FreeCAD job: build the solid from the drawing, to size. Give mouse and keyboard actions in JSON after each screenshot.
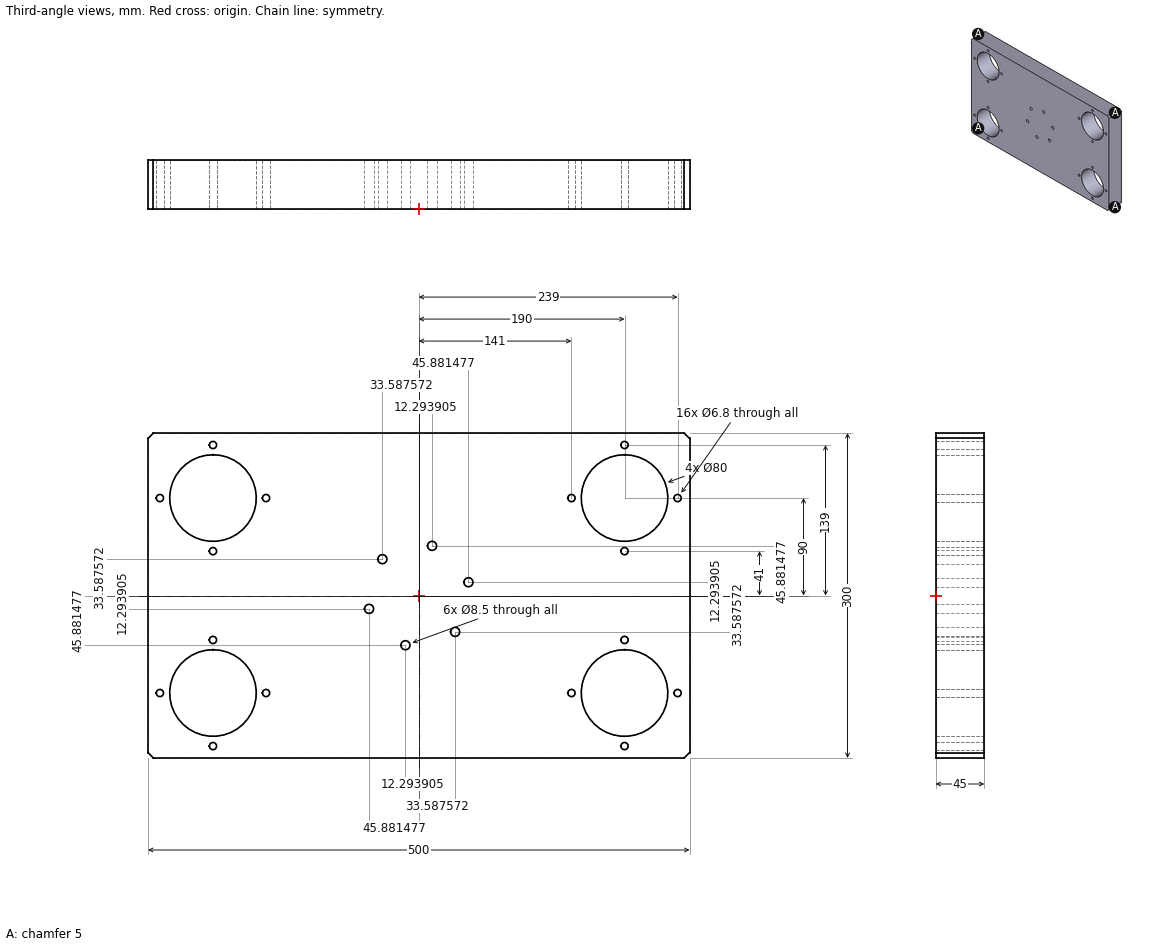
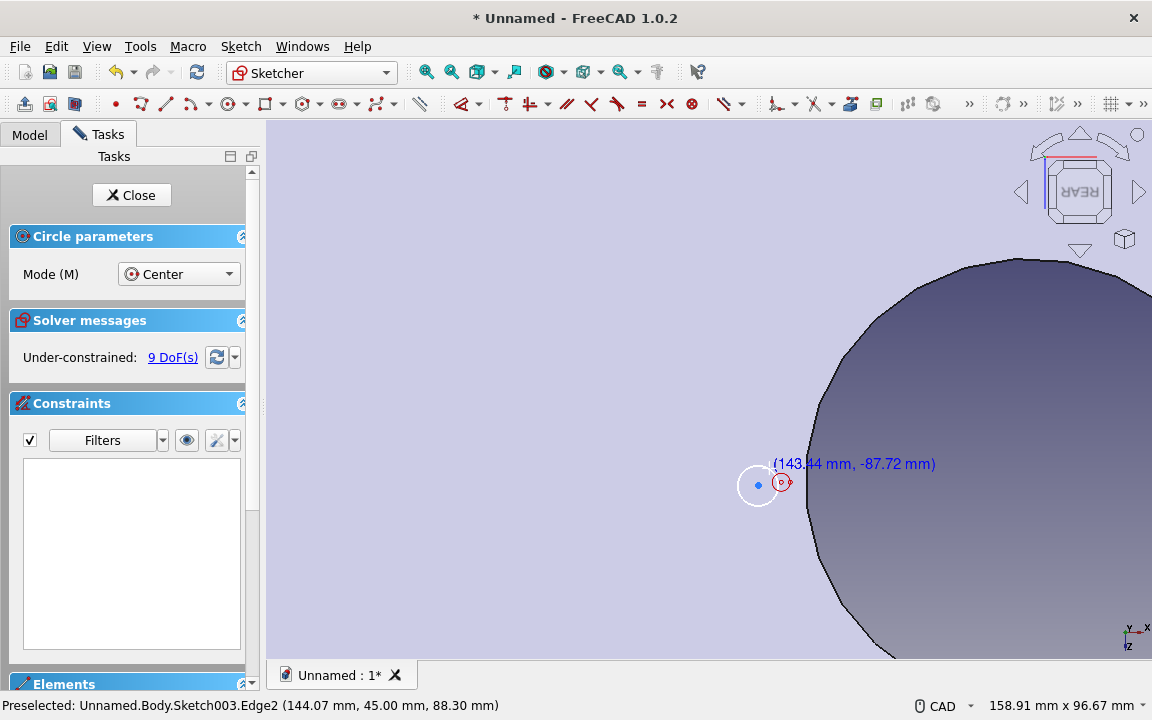
{"action": "scroll", "coordinate": [773, 471], "scroll_direction": "down", "scroll_amount": 9}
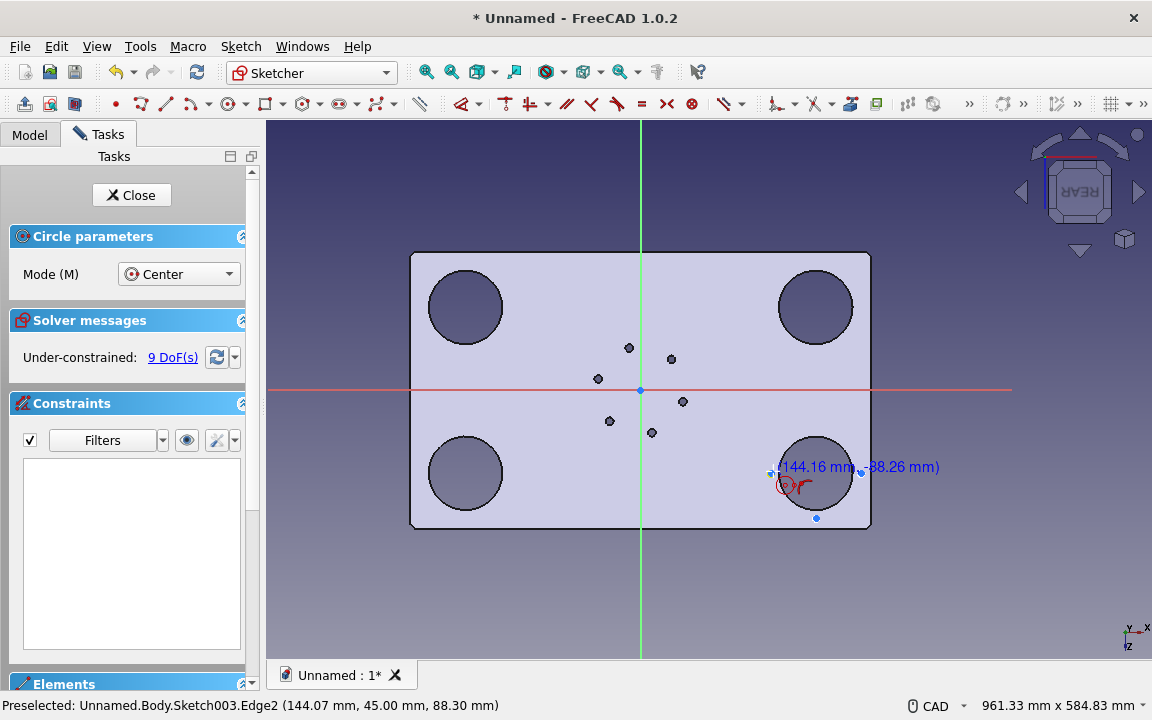
{"action": "scroll", "coordinate": [816, 428], "scroll_direction": "up", "scroll_amount": 10}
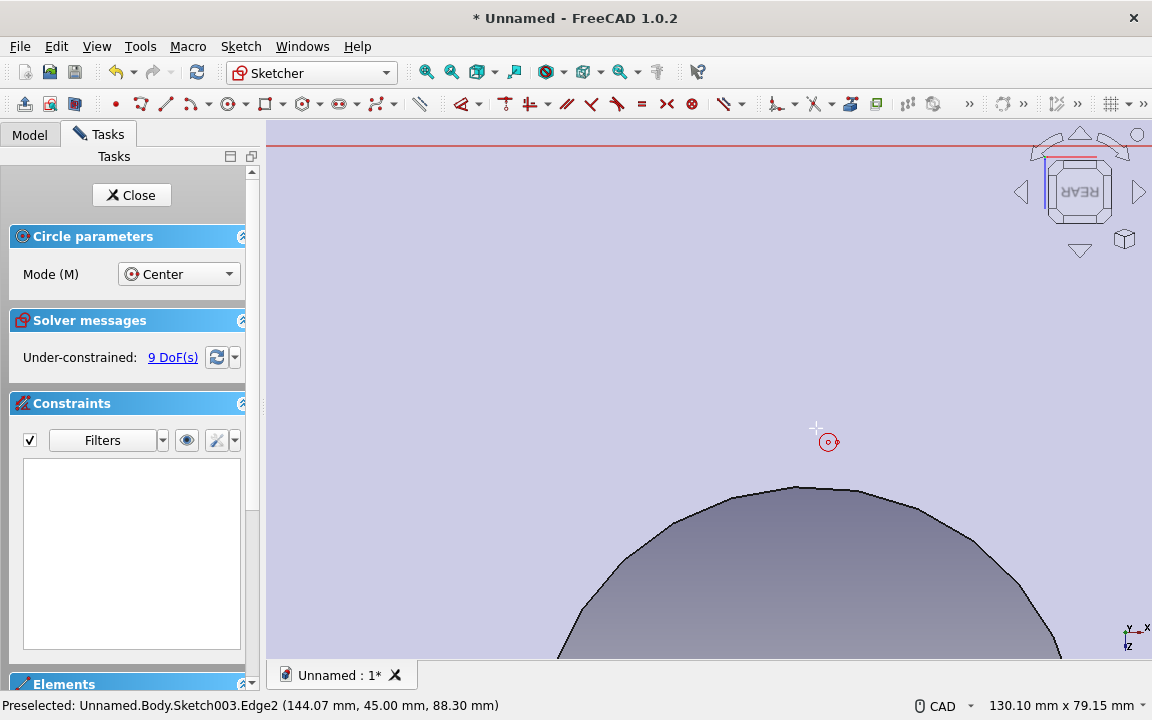
{"action": "scroll", "coordinate": [816, 428], "scroll_direction": "down", "scroll_amount": 10}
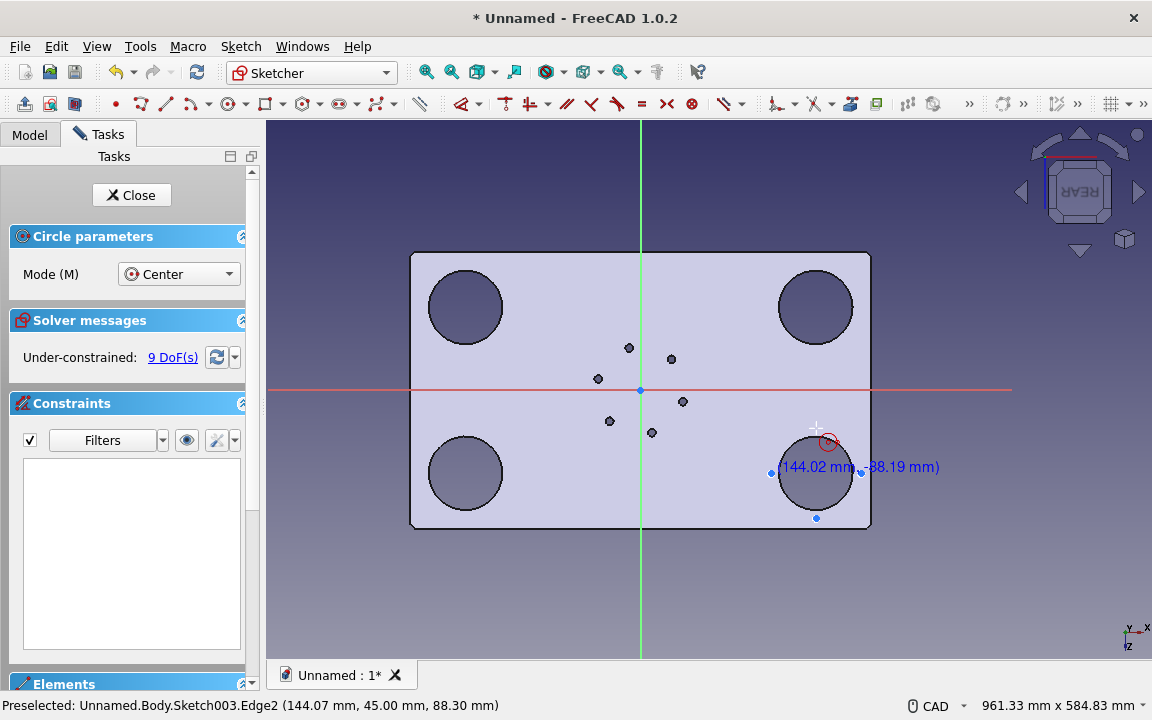
{"action": "left_click", "coordinate": [816, 428]}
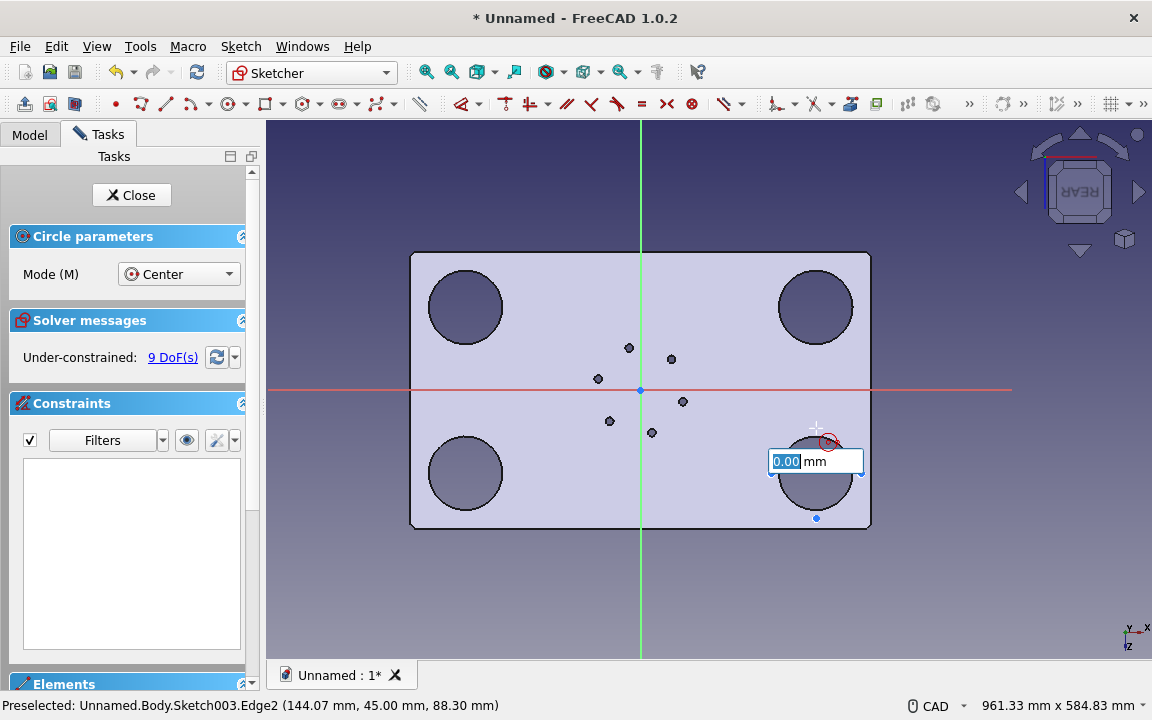
{"action": "scroll", "coordinate": [818, 426], "scroll_direction": "up", "scroll_amount": 9}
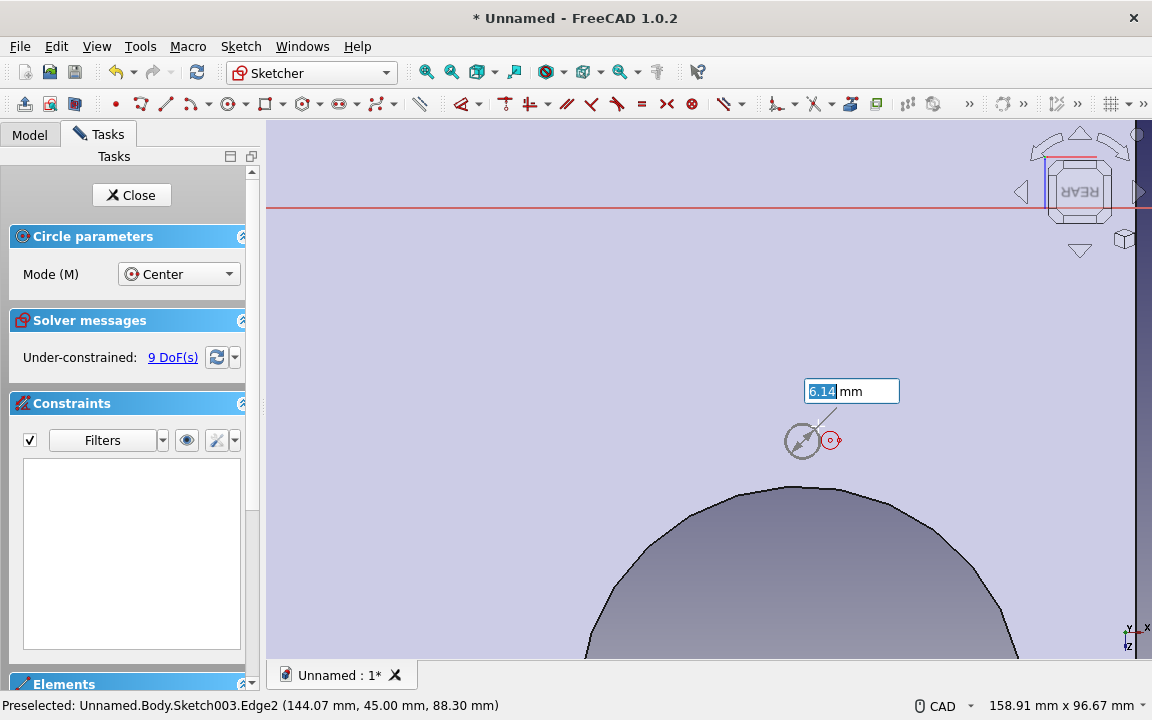
{"action": "left_click", "coordinate": [814, 423]}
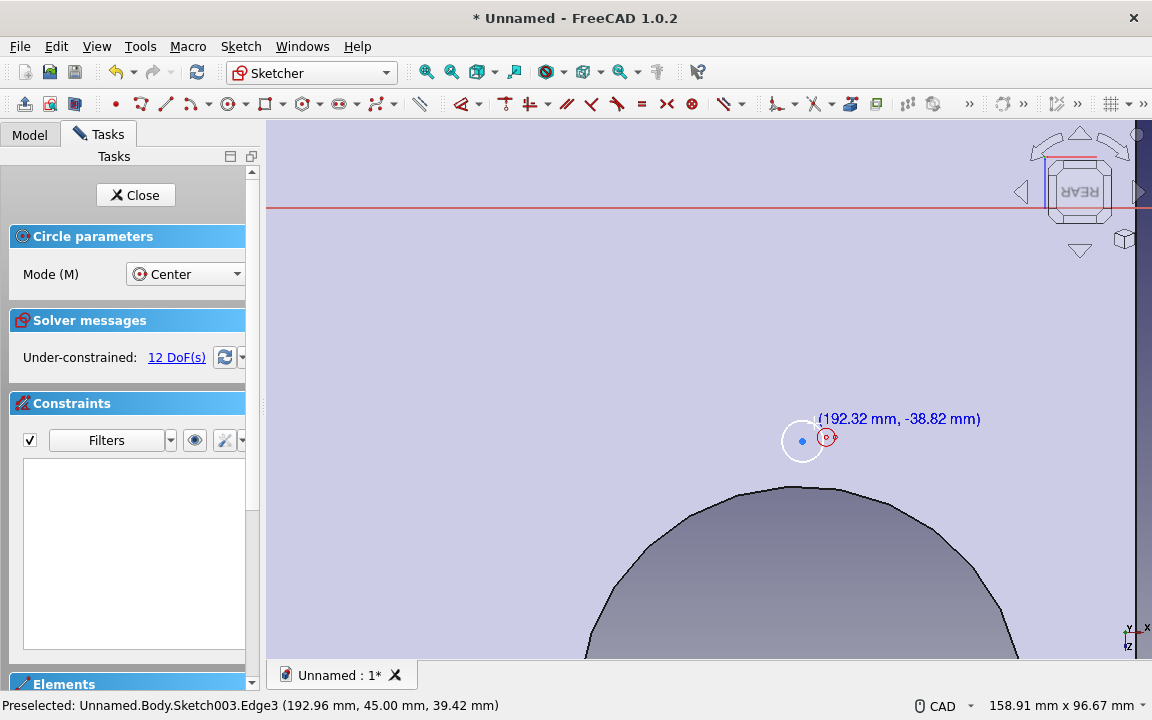
{"action": "scroll", "coordinate": [818, 426], "scroll_direction": "down", "scroll_amount": 9}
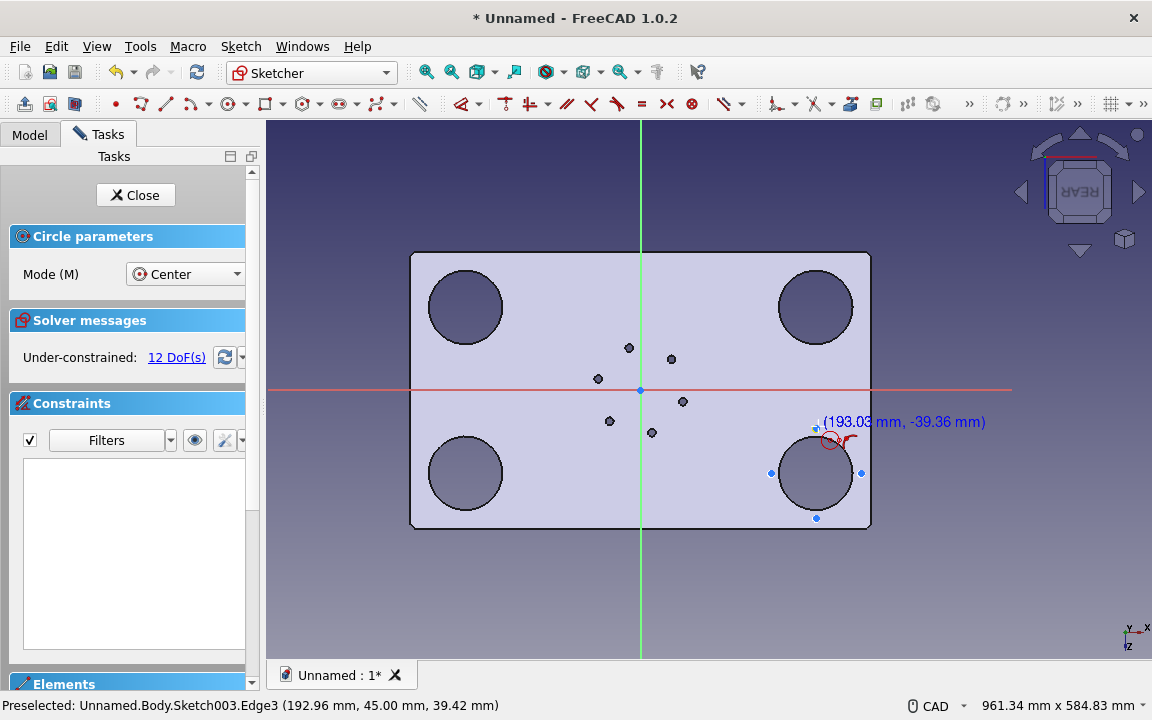
{"action": "scroll", "coordinate": [861, 307], "scroll_direction": "up", "scroll_amount": 10}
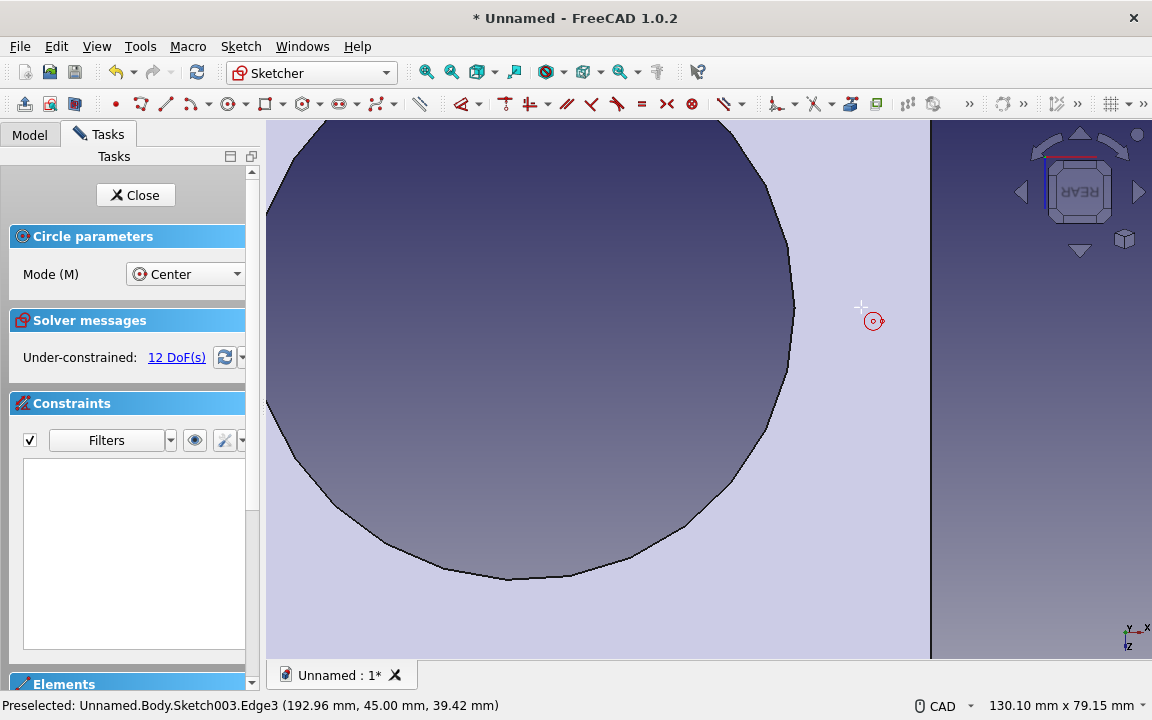
{"action": "scroll", "coordinate": [862, 306], "scroll_direction": "down", "scroll_amount": 10}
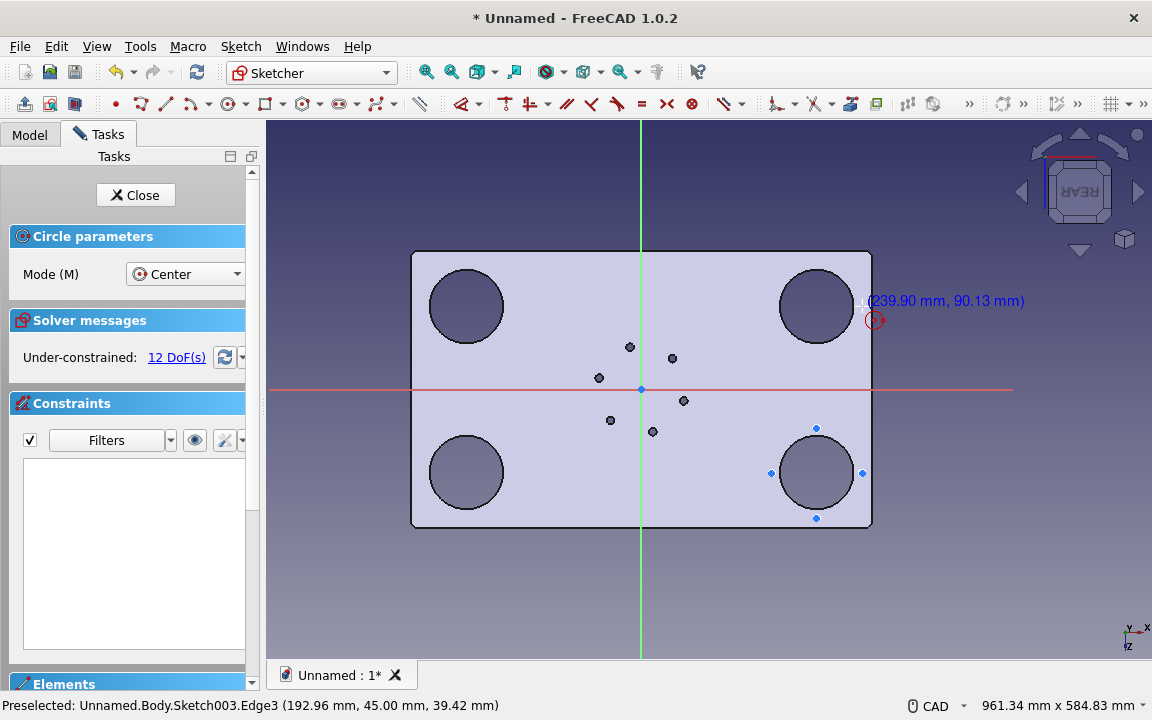
{"action": "left_click", "coordinate": [862, 307]}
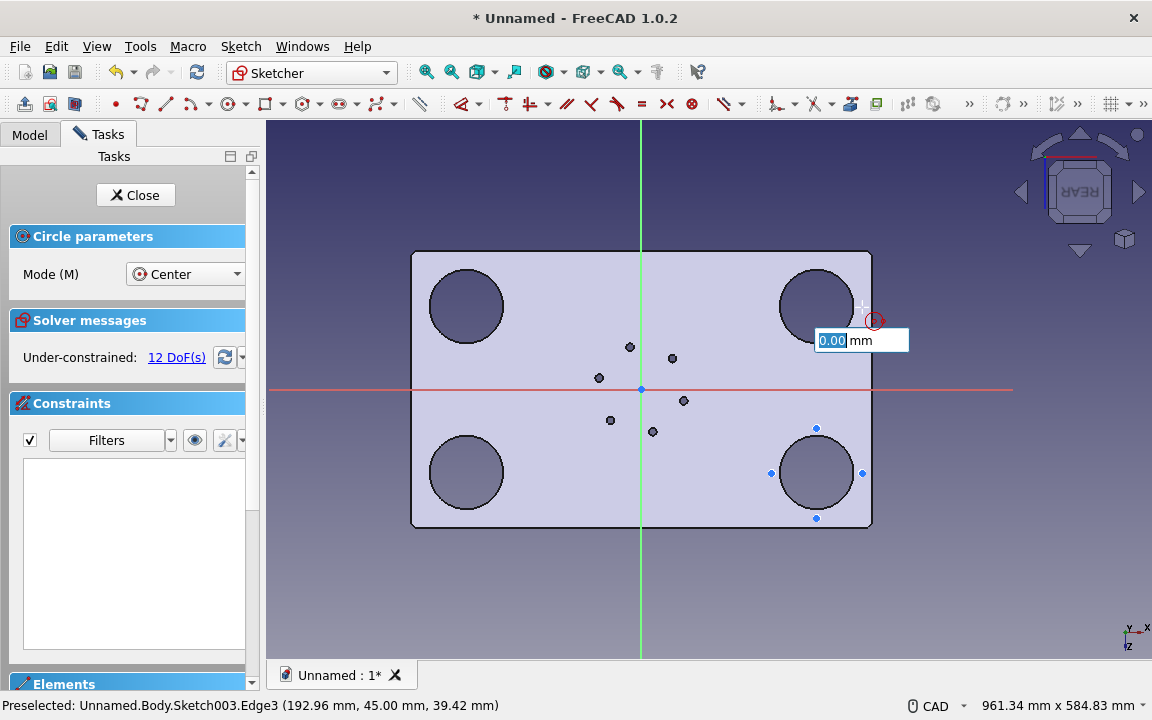
{"action": "scroll", "coordinate": [864, 304], "scroll_direction": "up", "scroll_amount": 9}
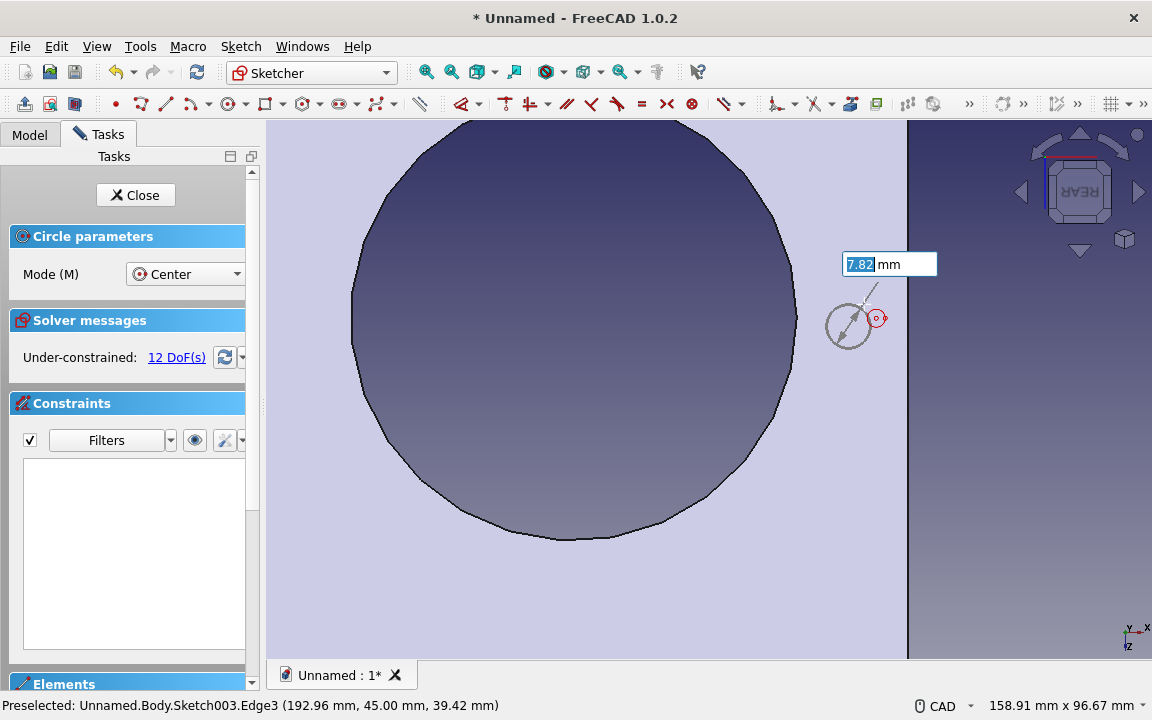
{"action": "left_click", "coordinate": [860, 304]}